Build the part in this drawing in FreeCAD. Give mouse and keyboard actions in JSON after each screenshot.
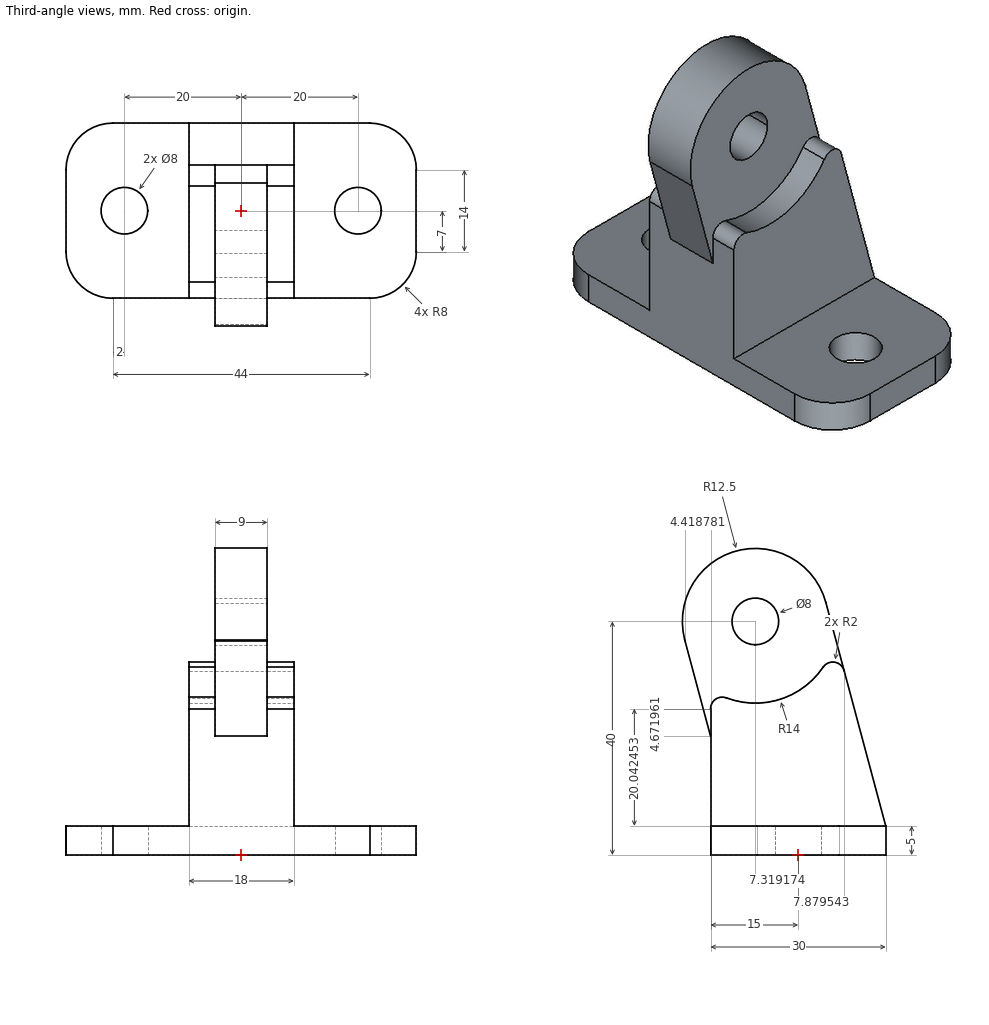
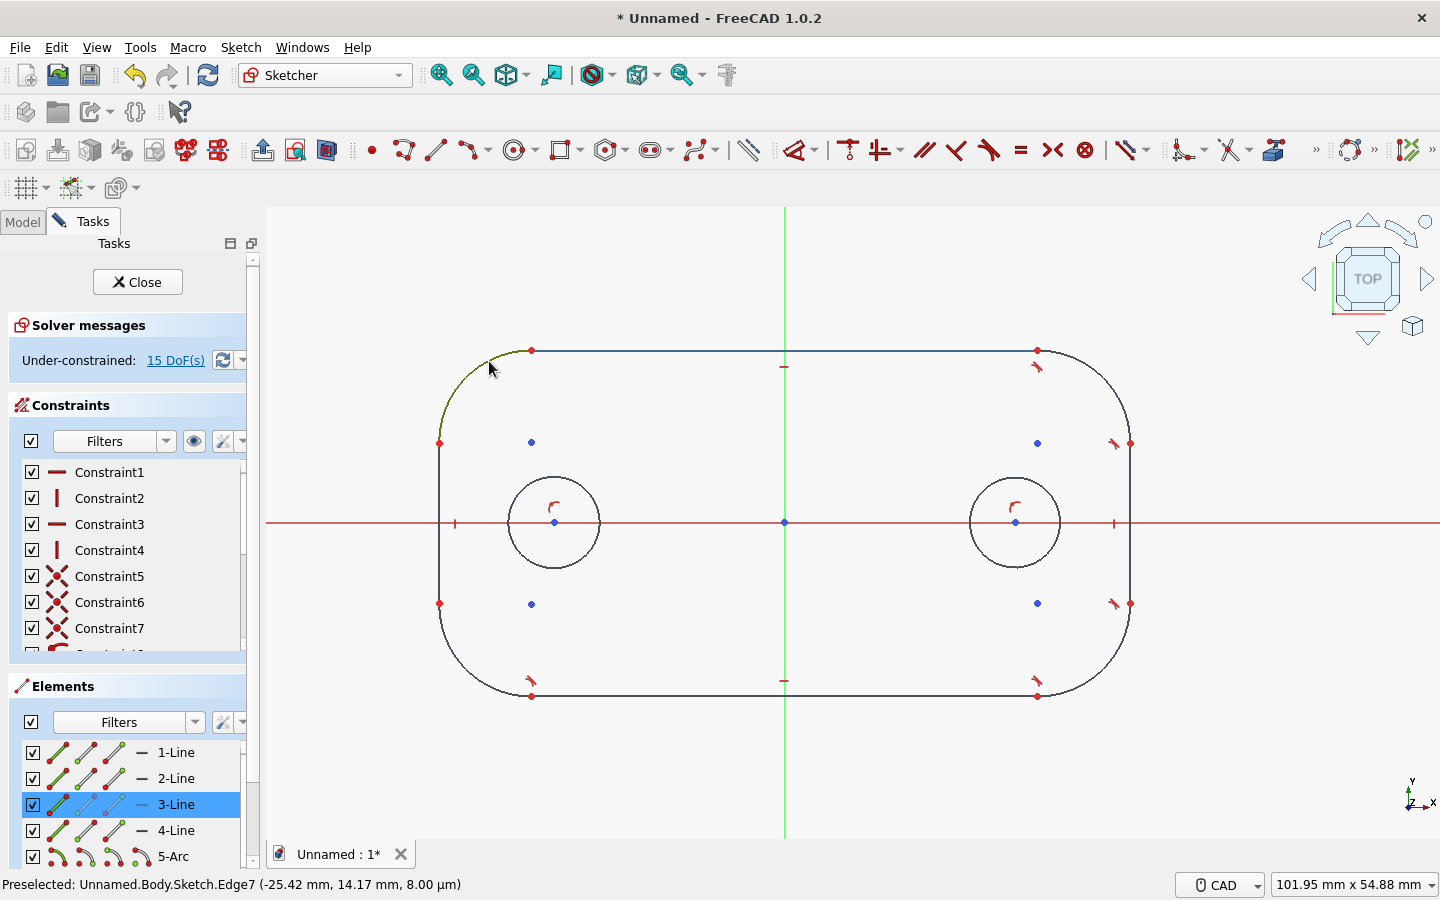
{"action": "key", "text": "t"}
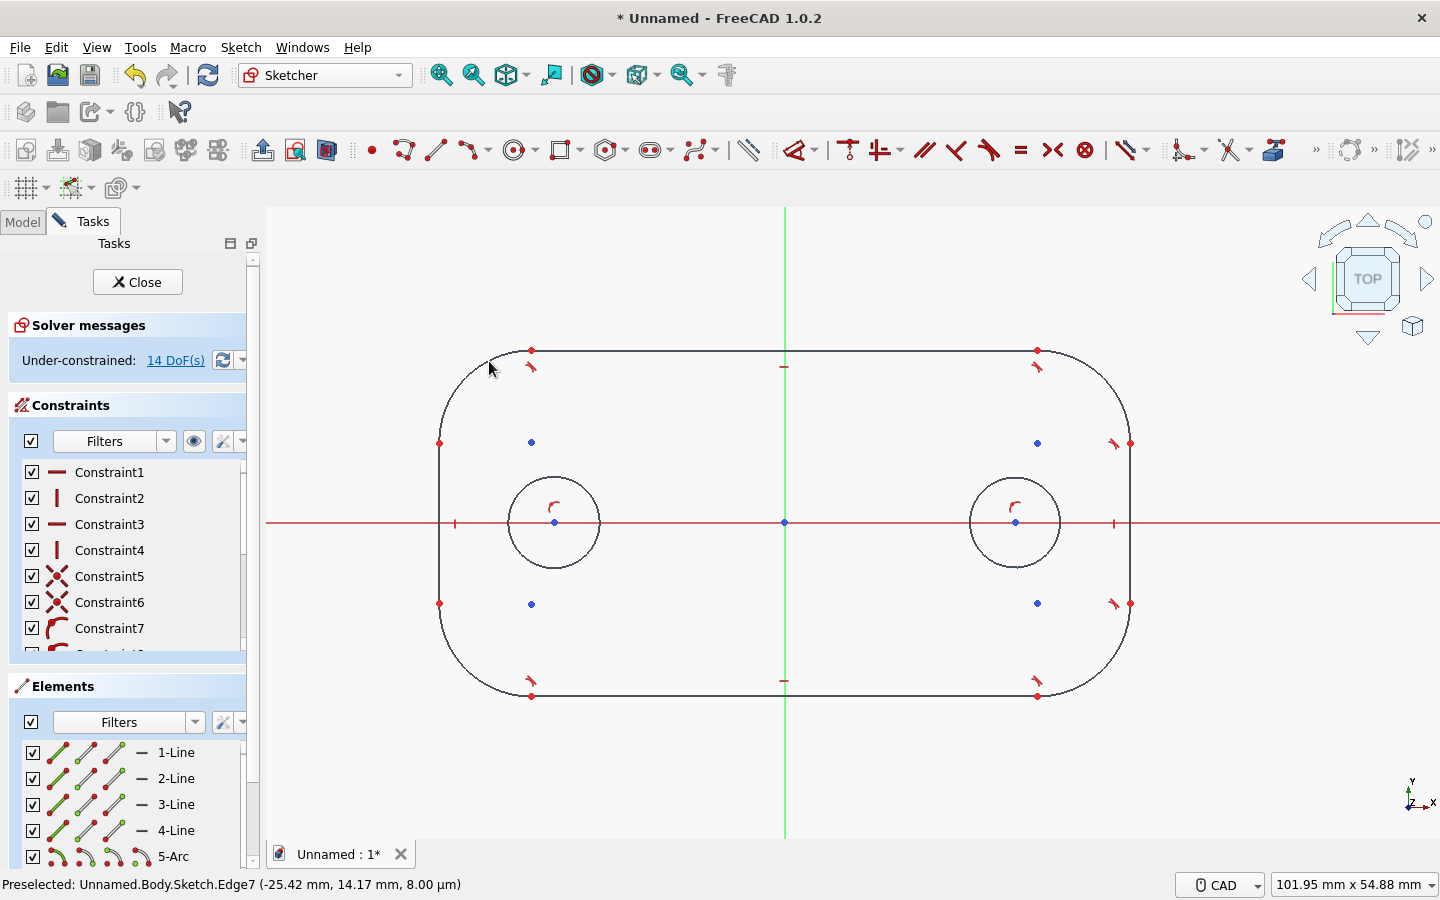
{"action": "left_click", "coordinate": [439, 491]}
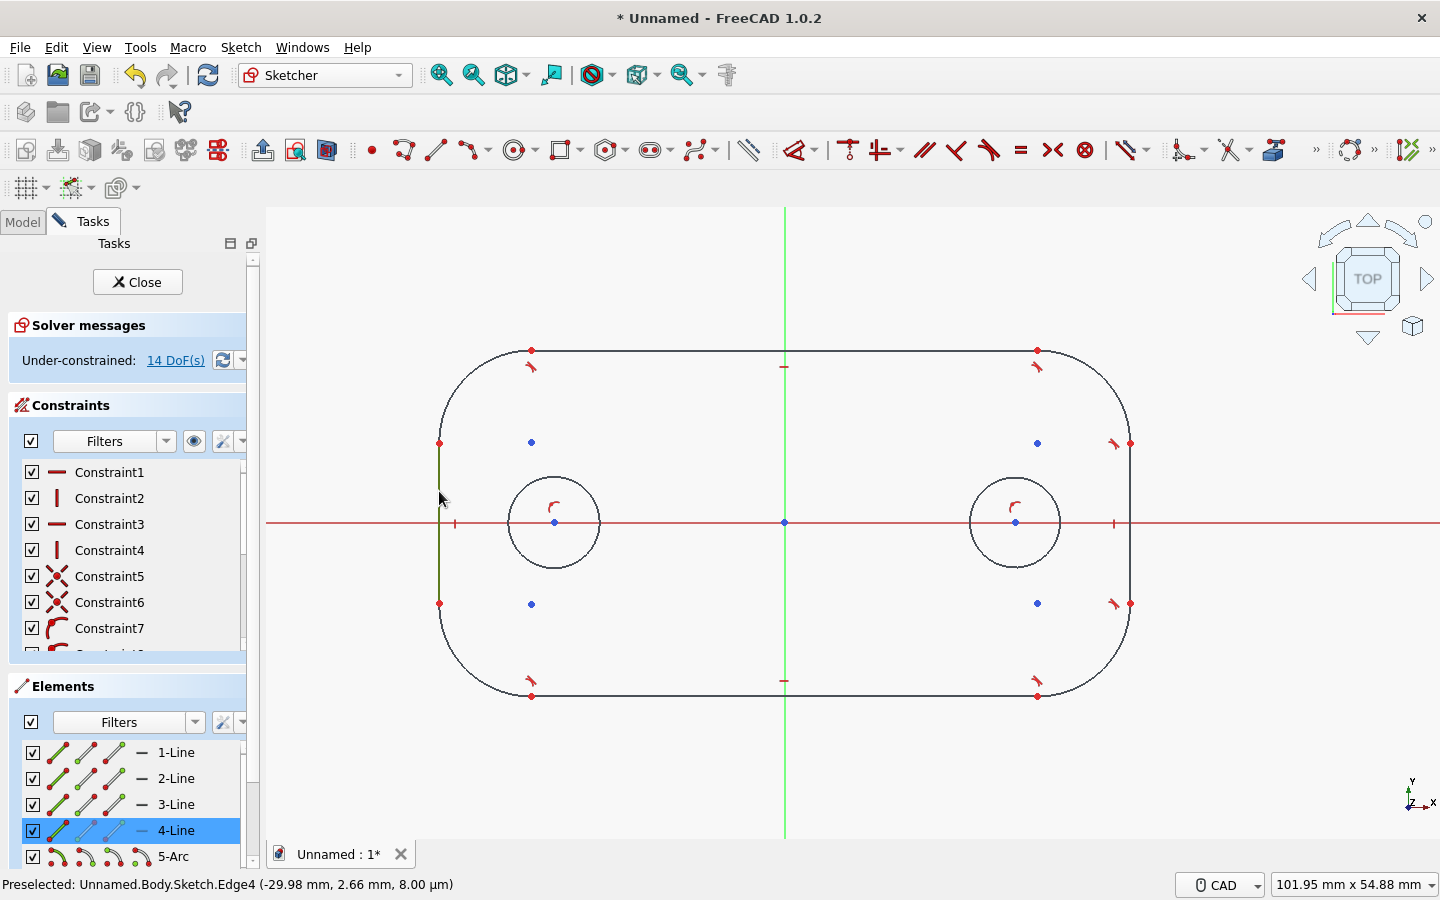
{"action": "left_click", "coordinate": [489, 361]}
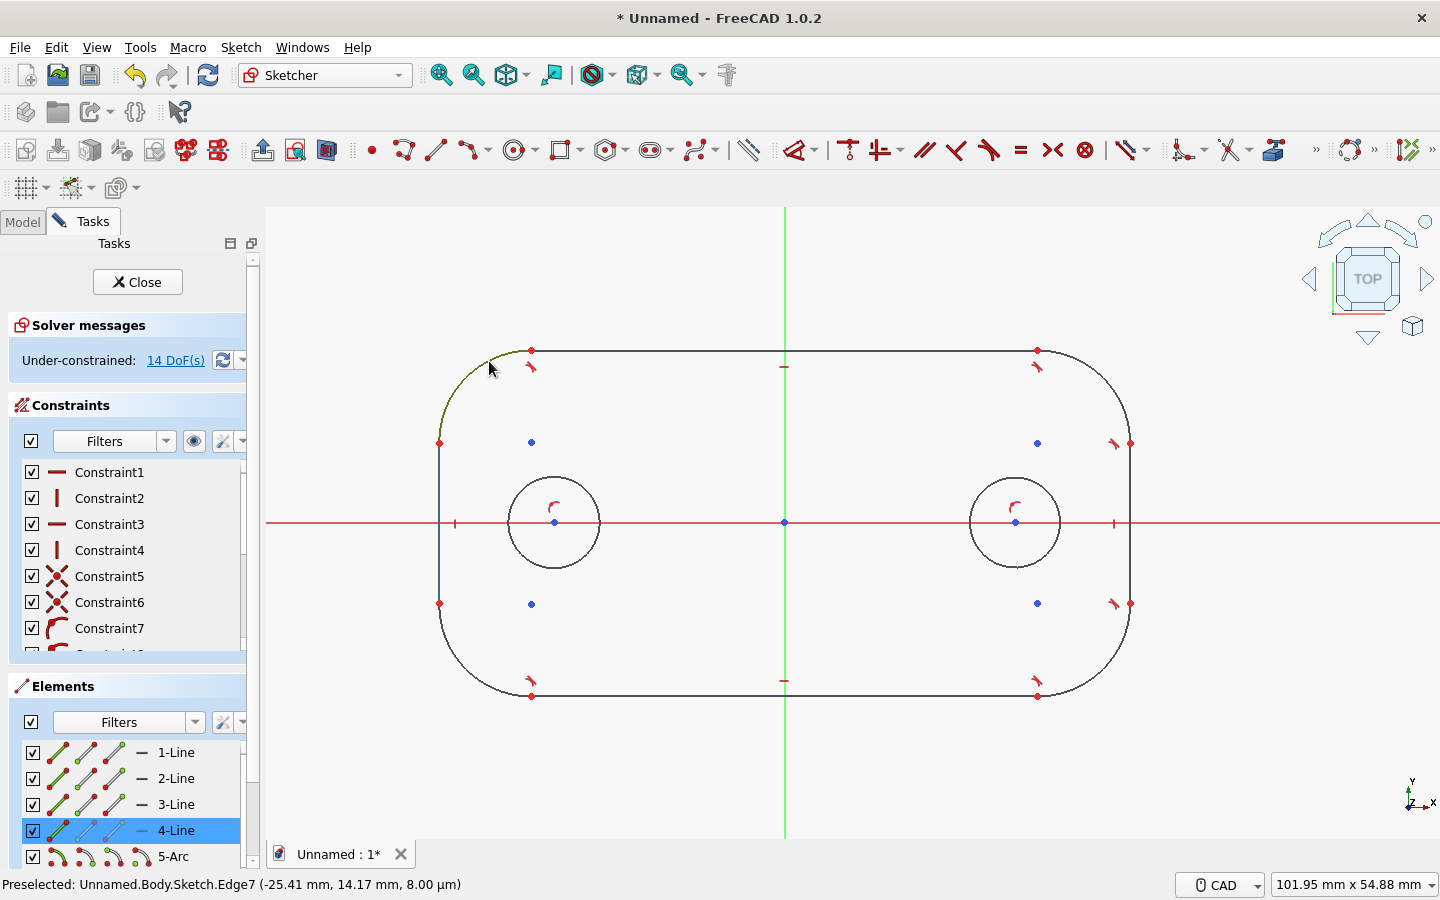
{"action": "key", "text": "t"}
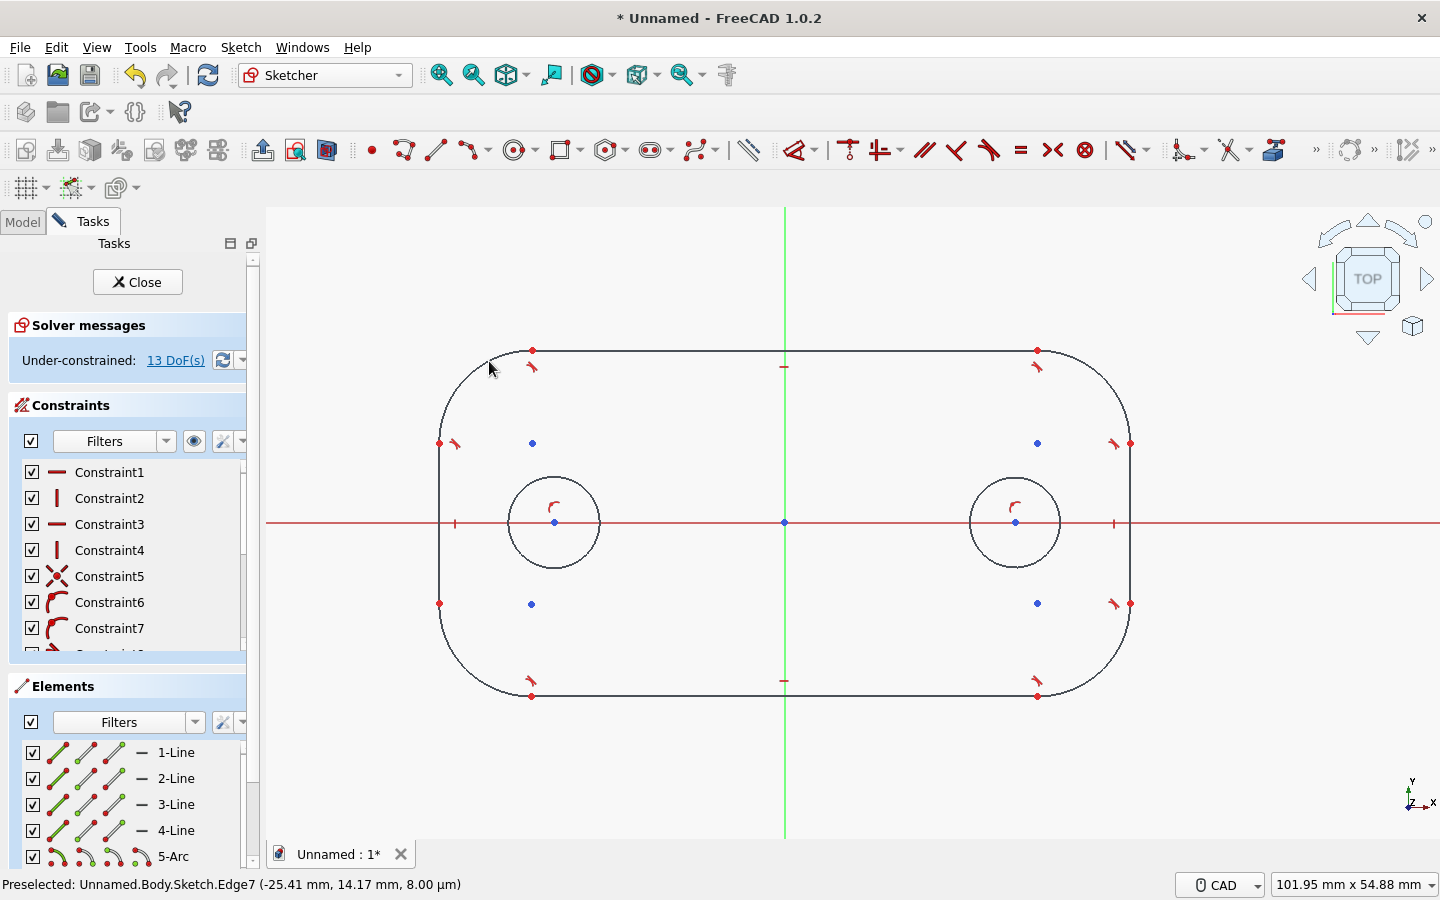
{"action": "left_click", "coordinate": [439, 491]}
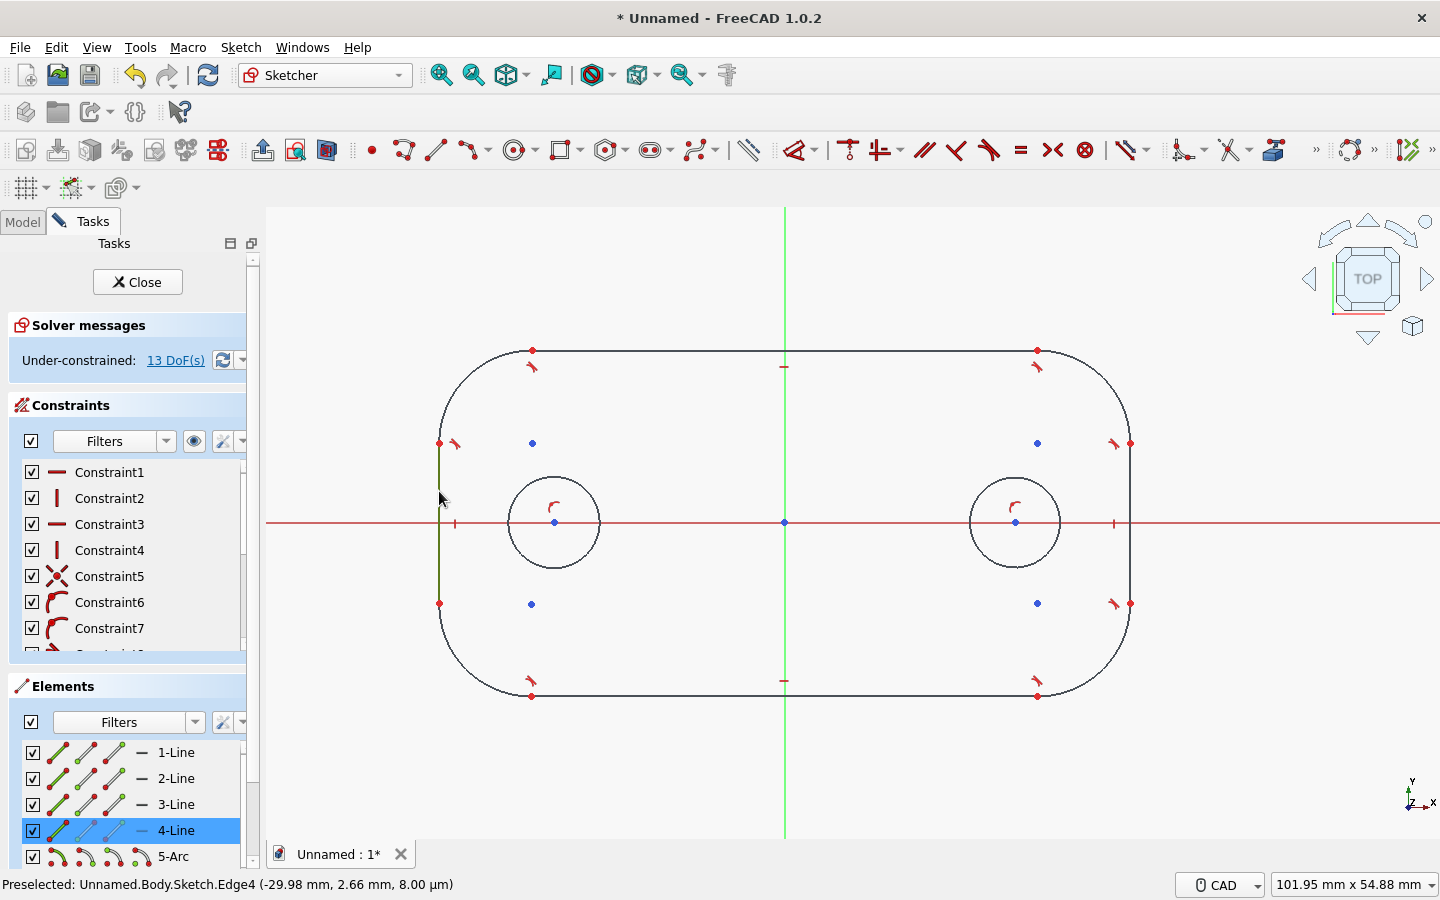
{"action": "left_click", "coordinate": [449, 646]}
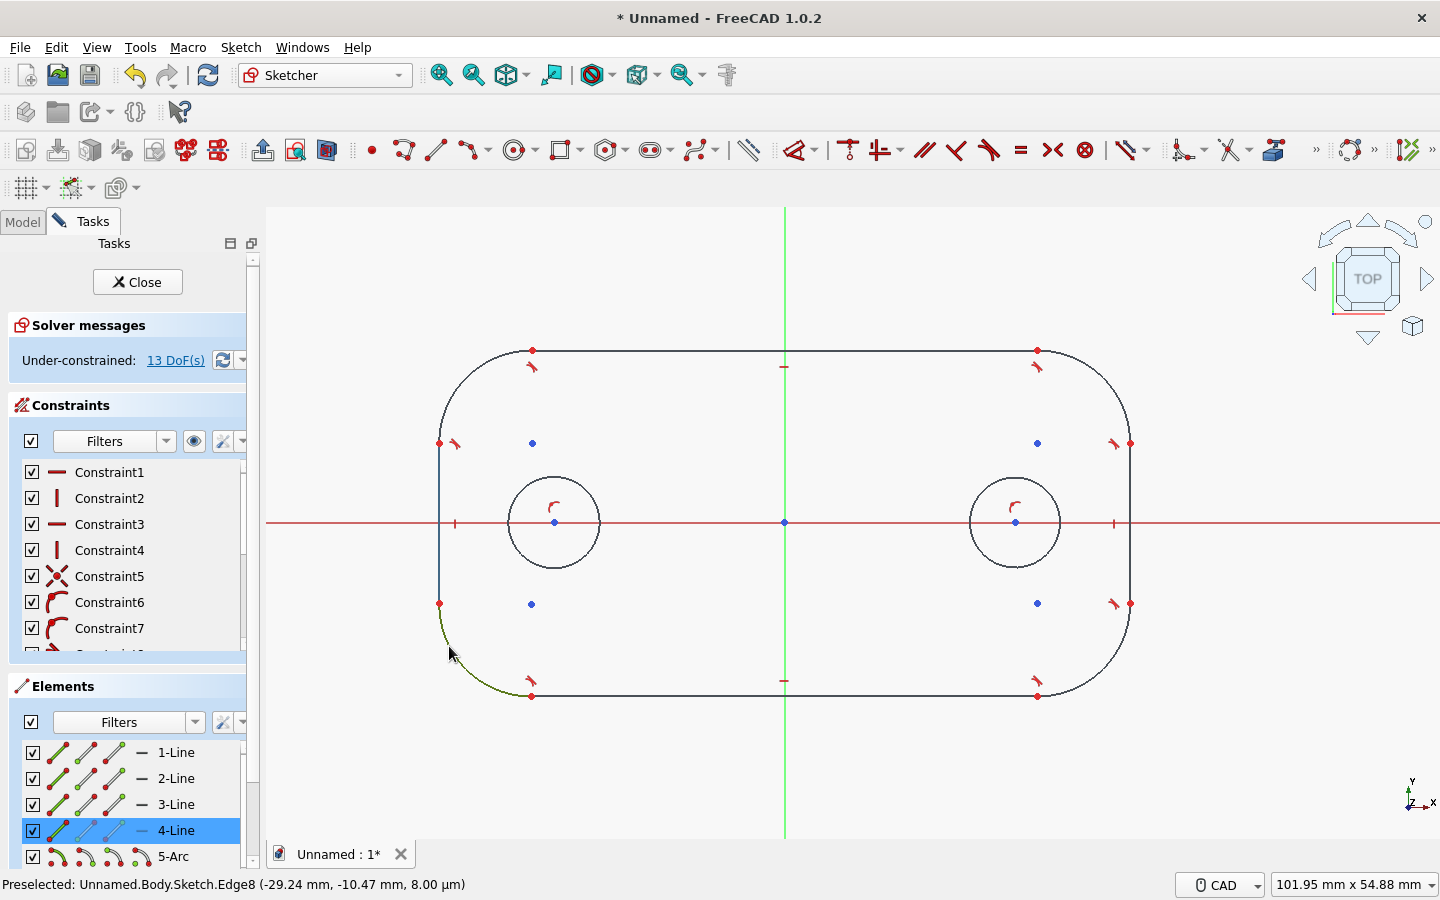
{"action": "key", "text": "t"}